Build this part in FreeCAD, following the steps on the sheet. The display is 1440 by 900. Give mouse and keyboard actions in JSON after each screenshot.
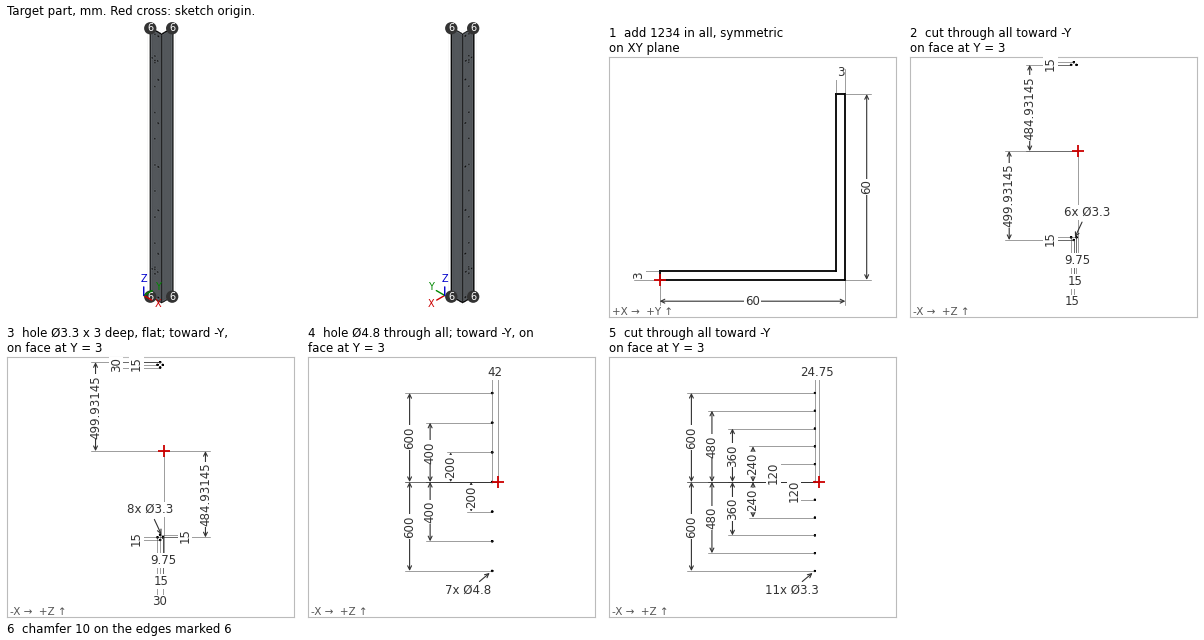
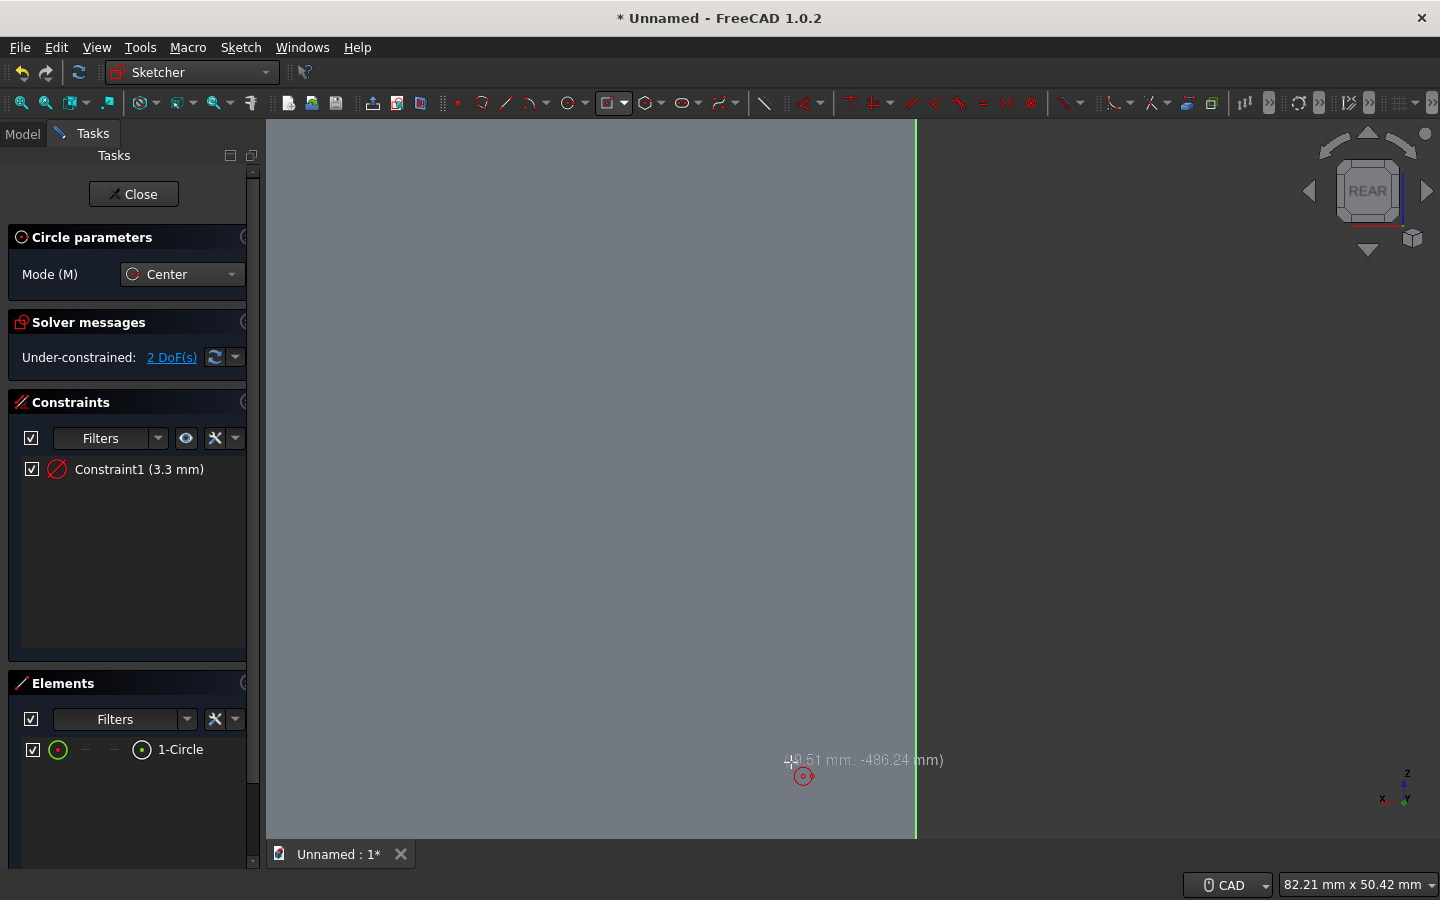
{"action": "scroll", "coordinate": [791, 762], "scroll_direction": "down", "scroll_amount": 16}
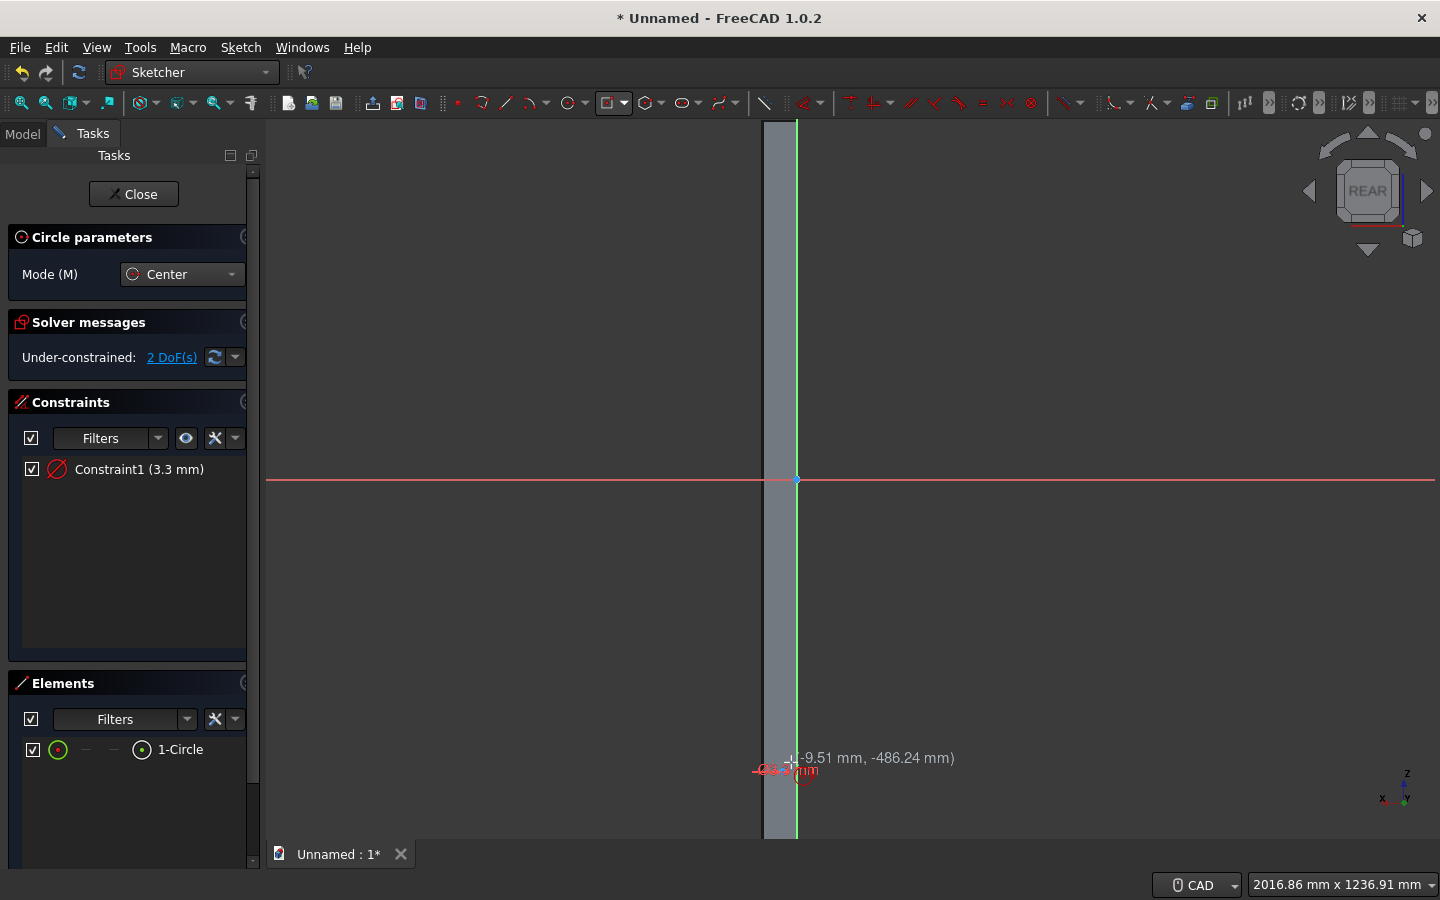
{"action": "scroll", "coordinate": [791, 762], "scroll_direction": "up", "scroll_amount": 6}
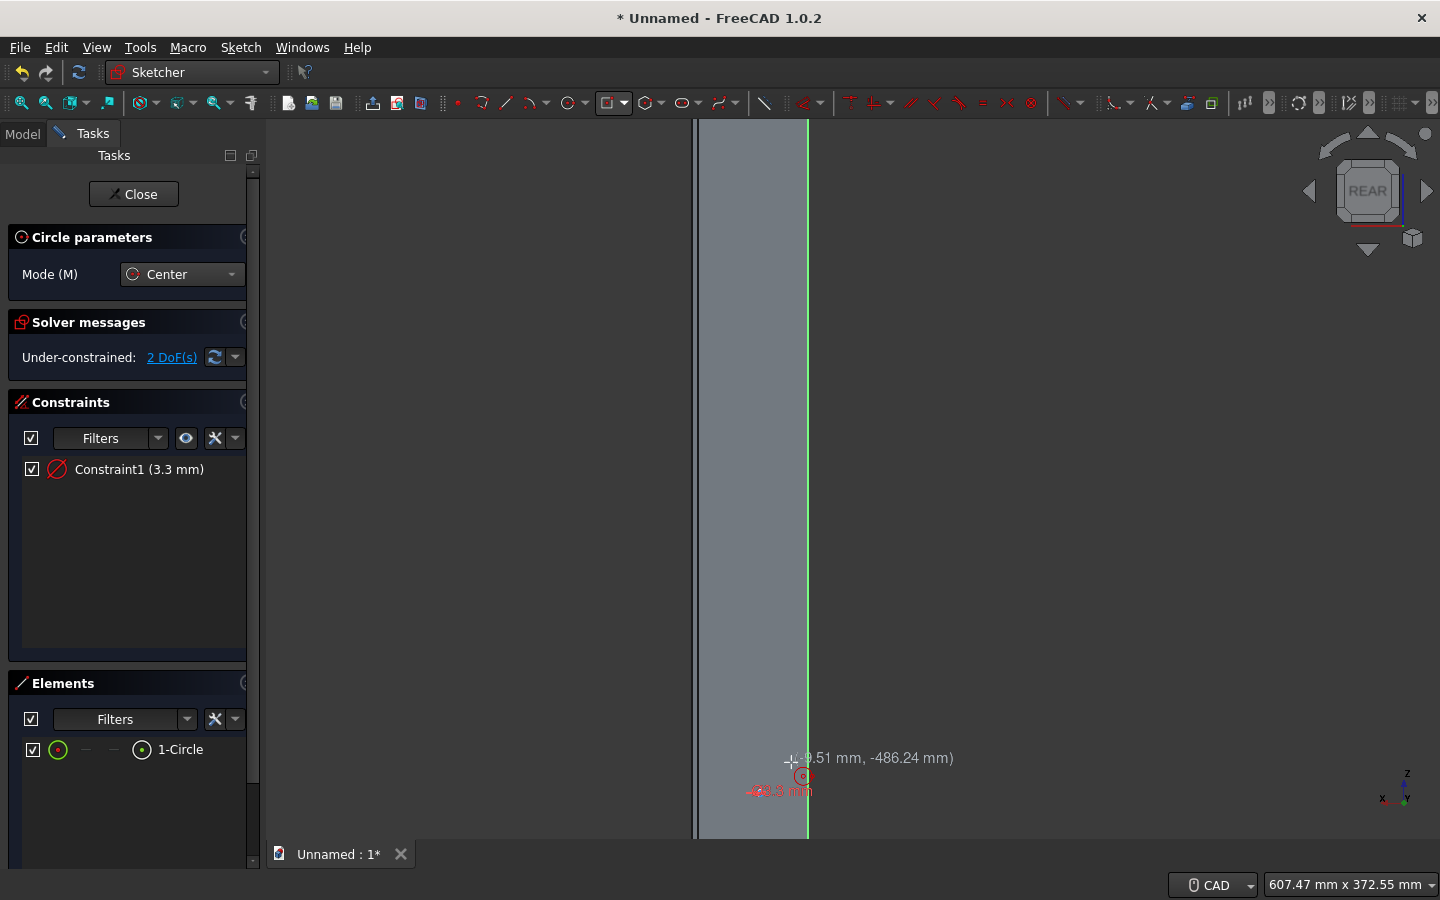
{"action": "left_click", "coordinate": [790, 761]}
{"action": "mouse_move", "coordinate": [792, 758]}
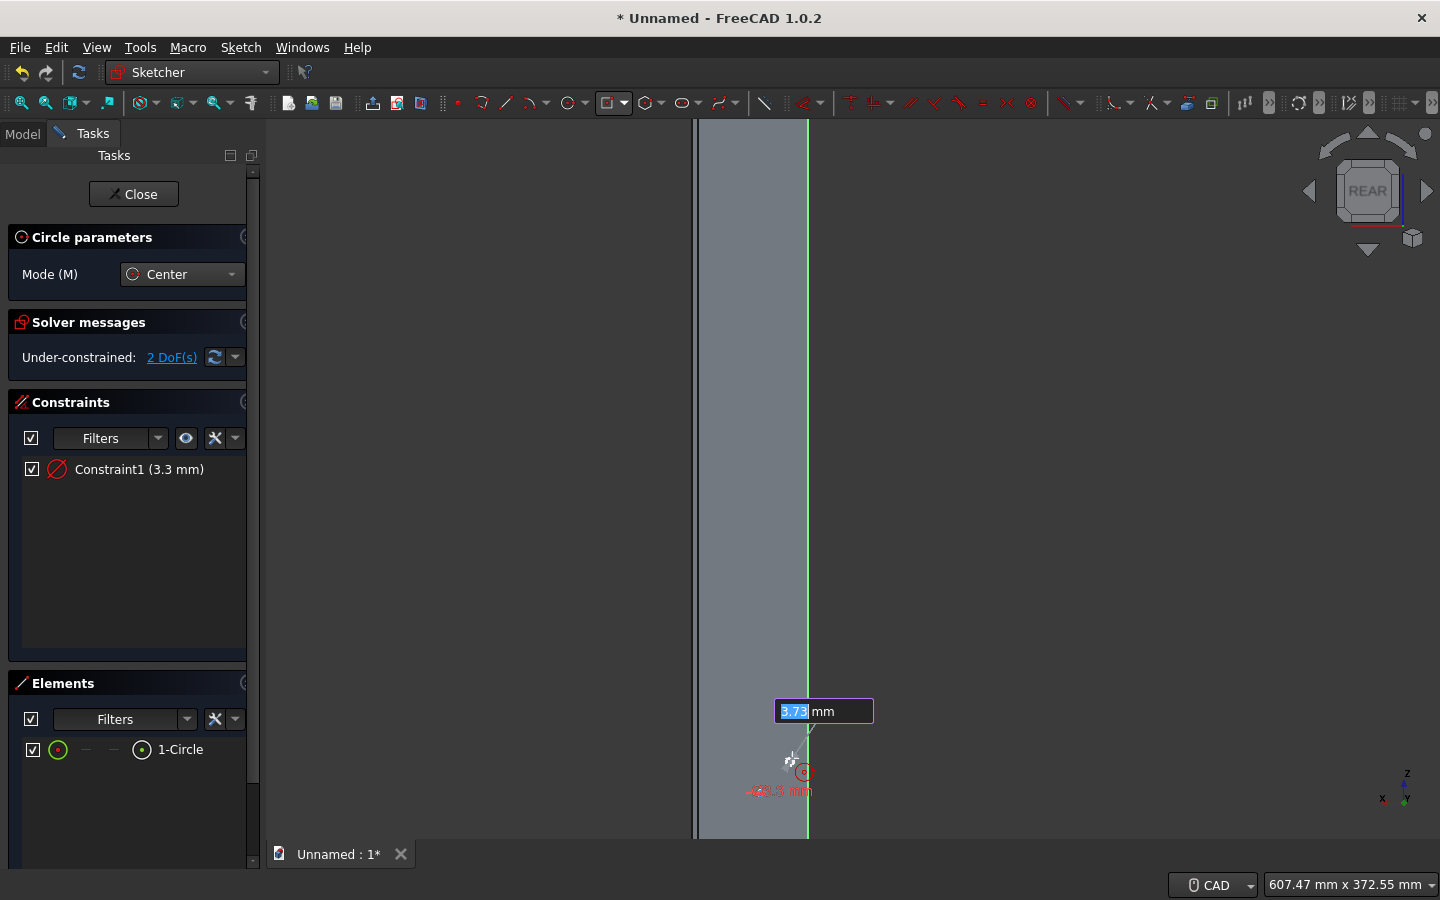
{"action": "type", "text": "3.3"}
{"action": "key", "text": "Return"}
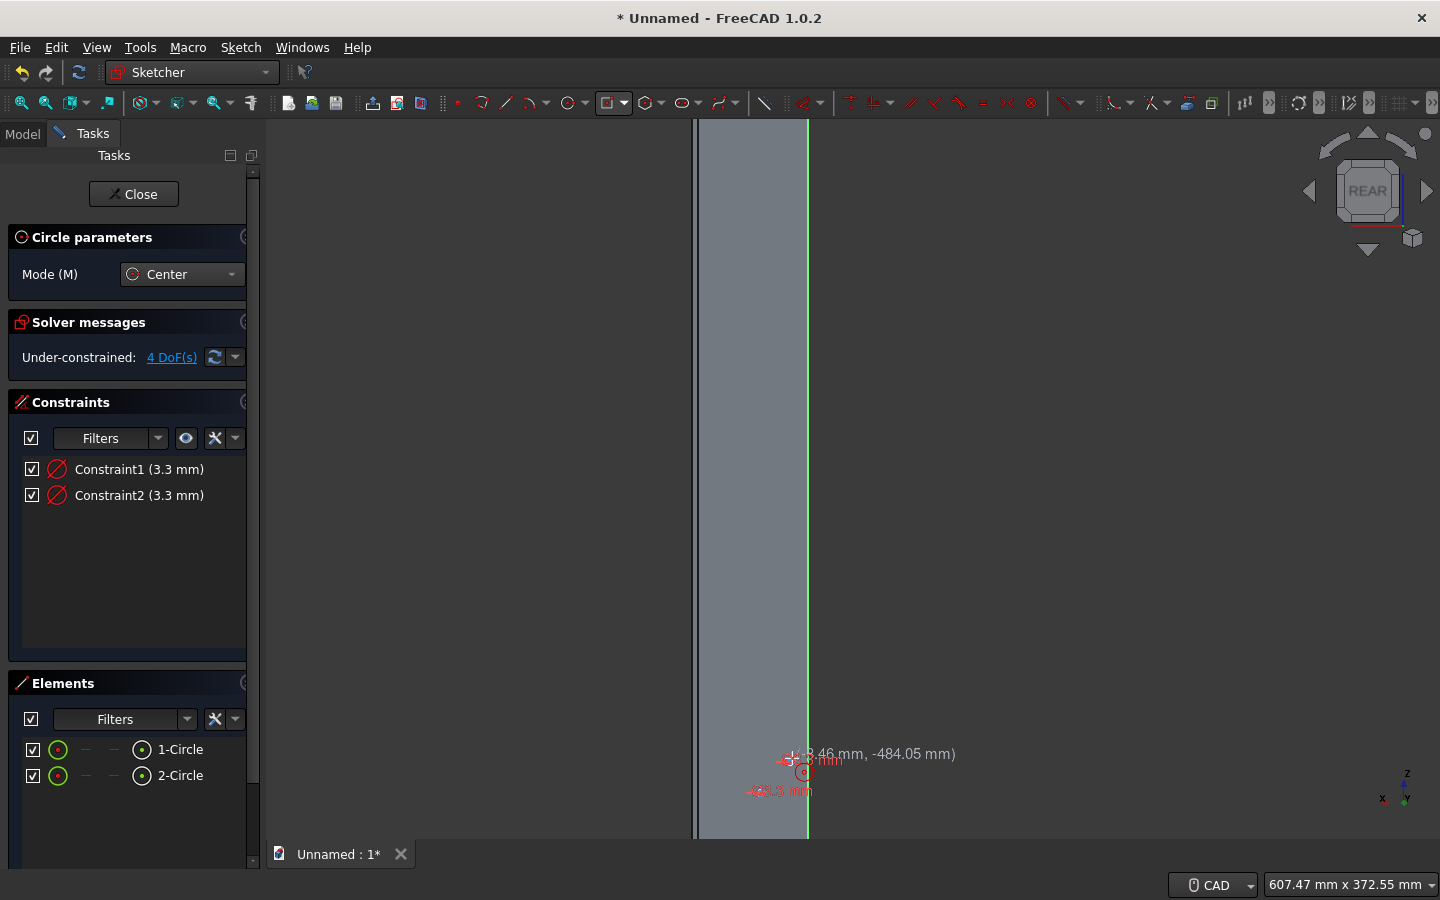
{"action": "scroll", "coordinate": [732, 761], "scroll_direction": "up", "scroll_amount": 10}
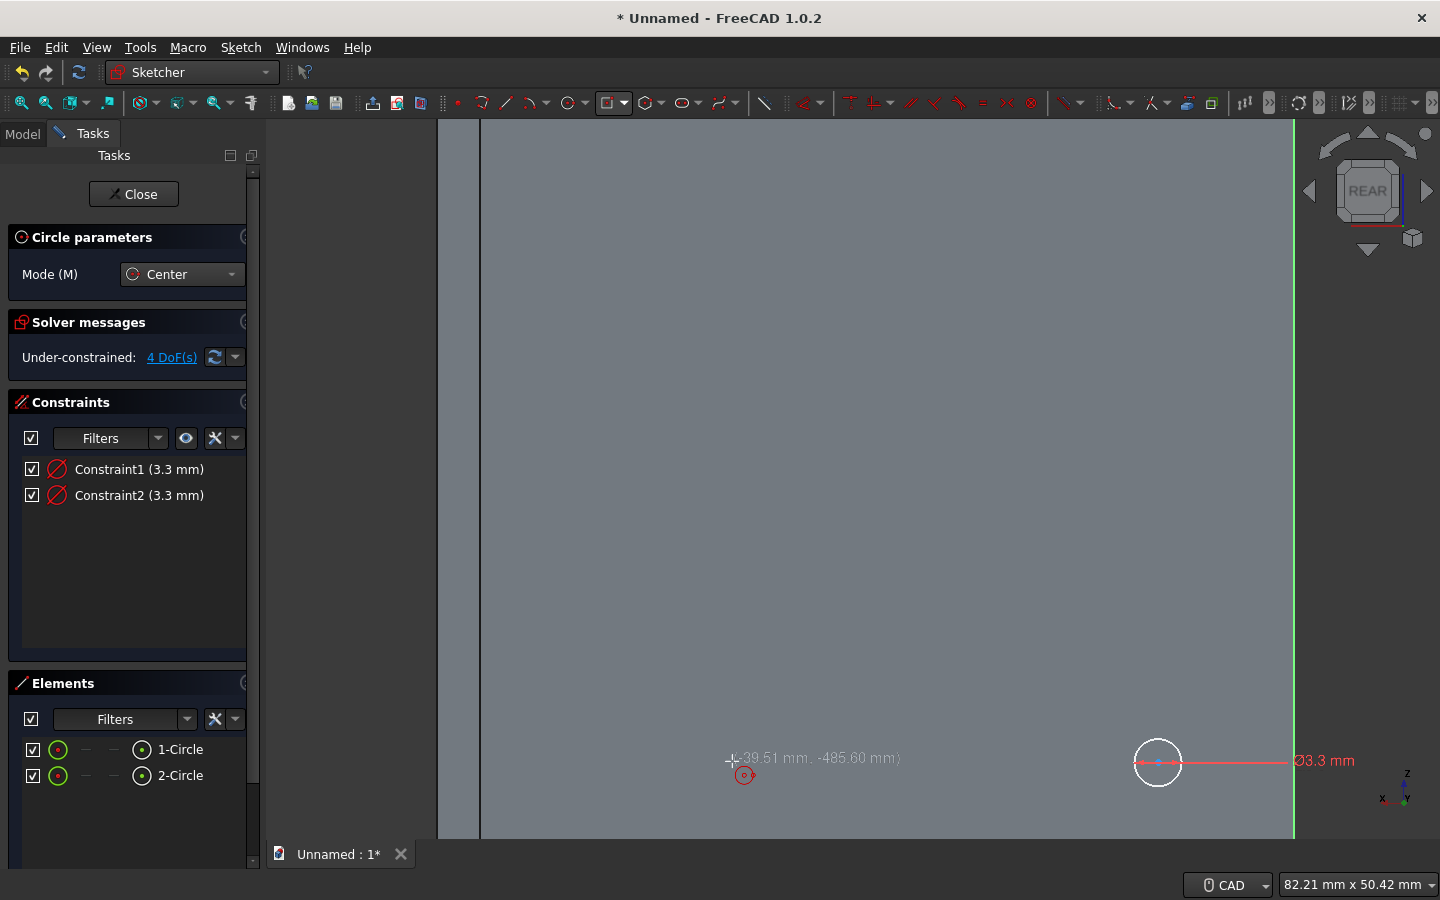
{"action": "scroll", "coordinate": [775, 762], "scroll_direction": "down", "scroll_amount": 16}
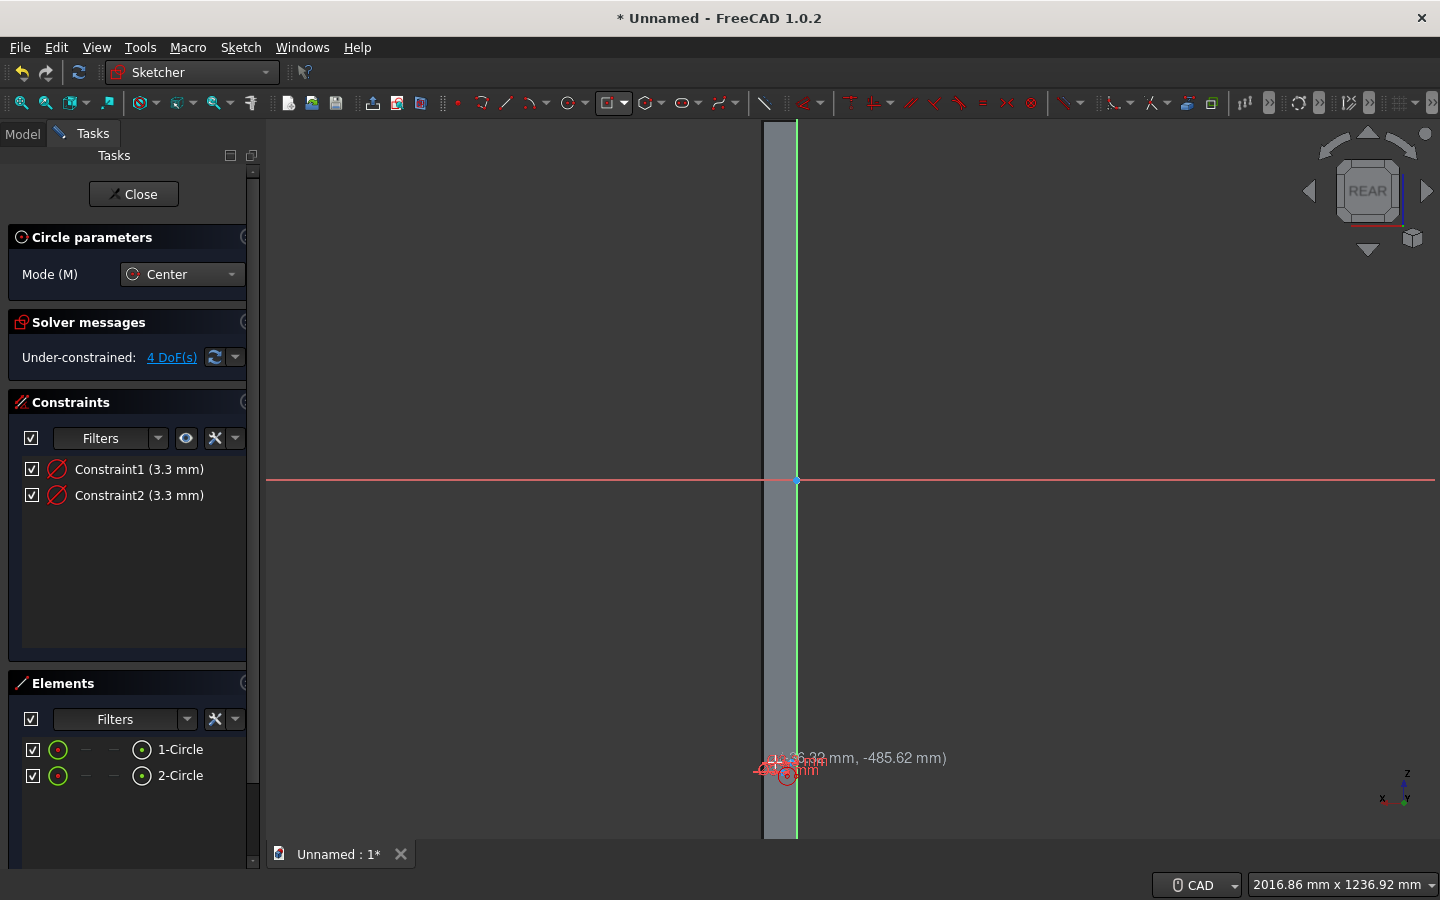
{"action": "scroll", "coordinate": [773, 762], "scroll_direction": "up", "scroll_amount": 2}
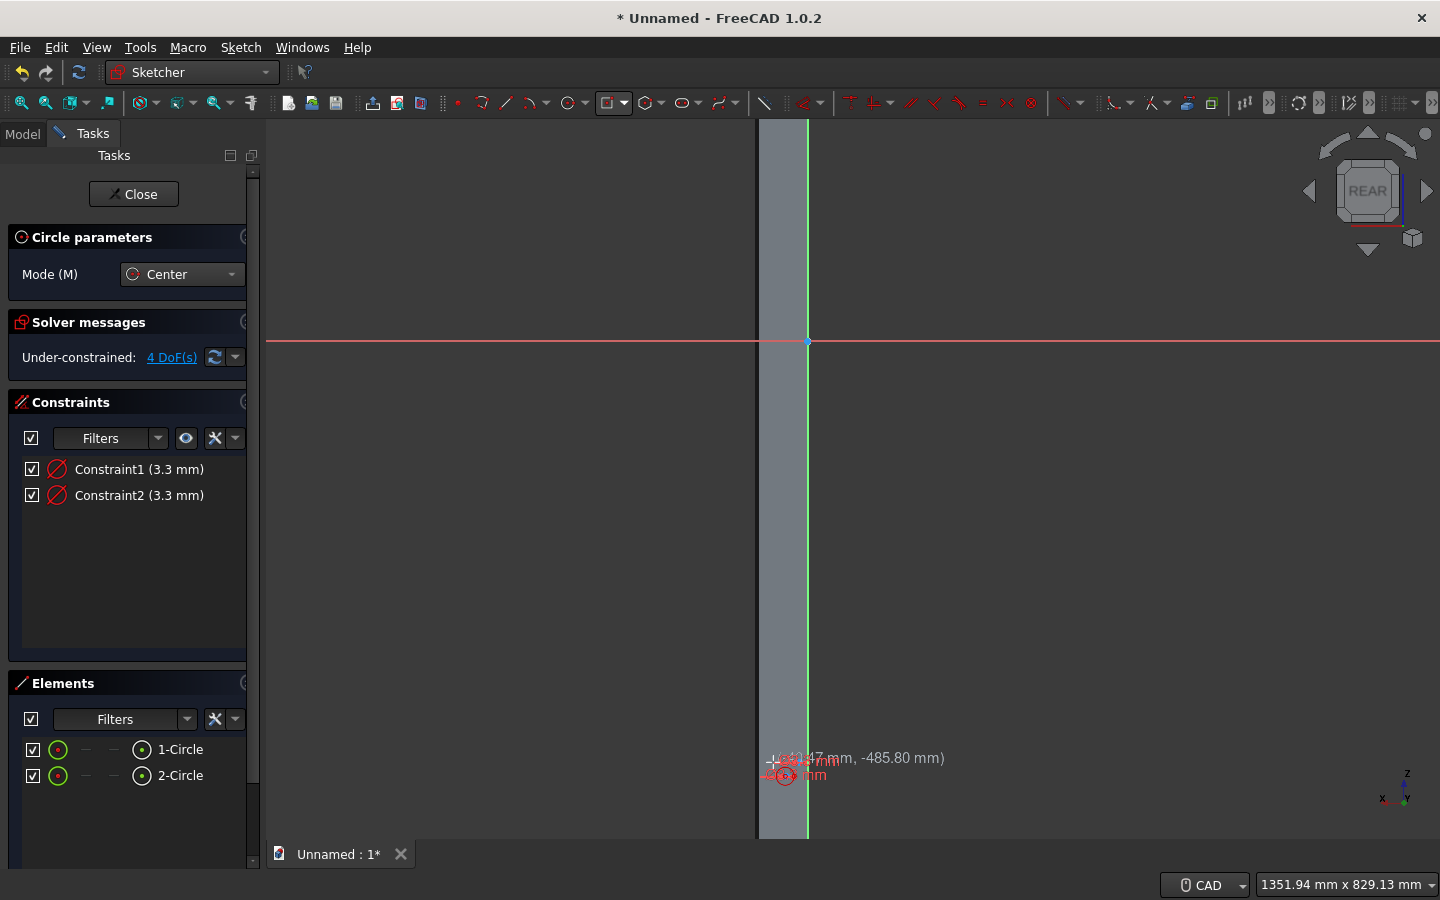
{"action": "left_click", "coordinate": [773, 762]}
{"action": "mouse_move", "coordinate": [774, 761]}